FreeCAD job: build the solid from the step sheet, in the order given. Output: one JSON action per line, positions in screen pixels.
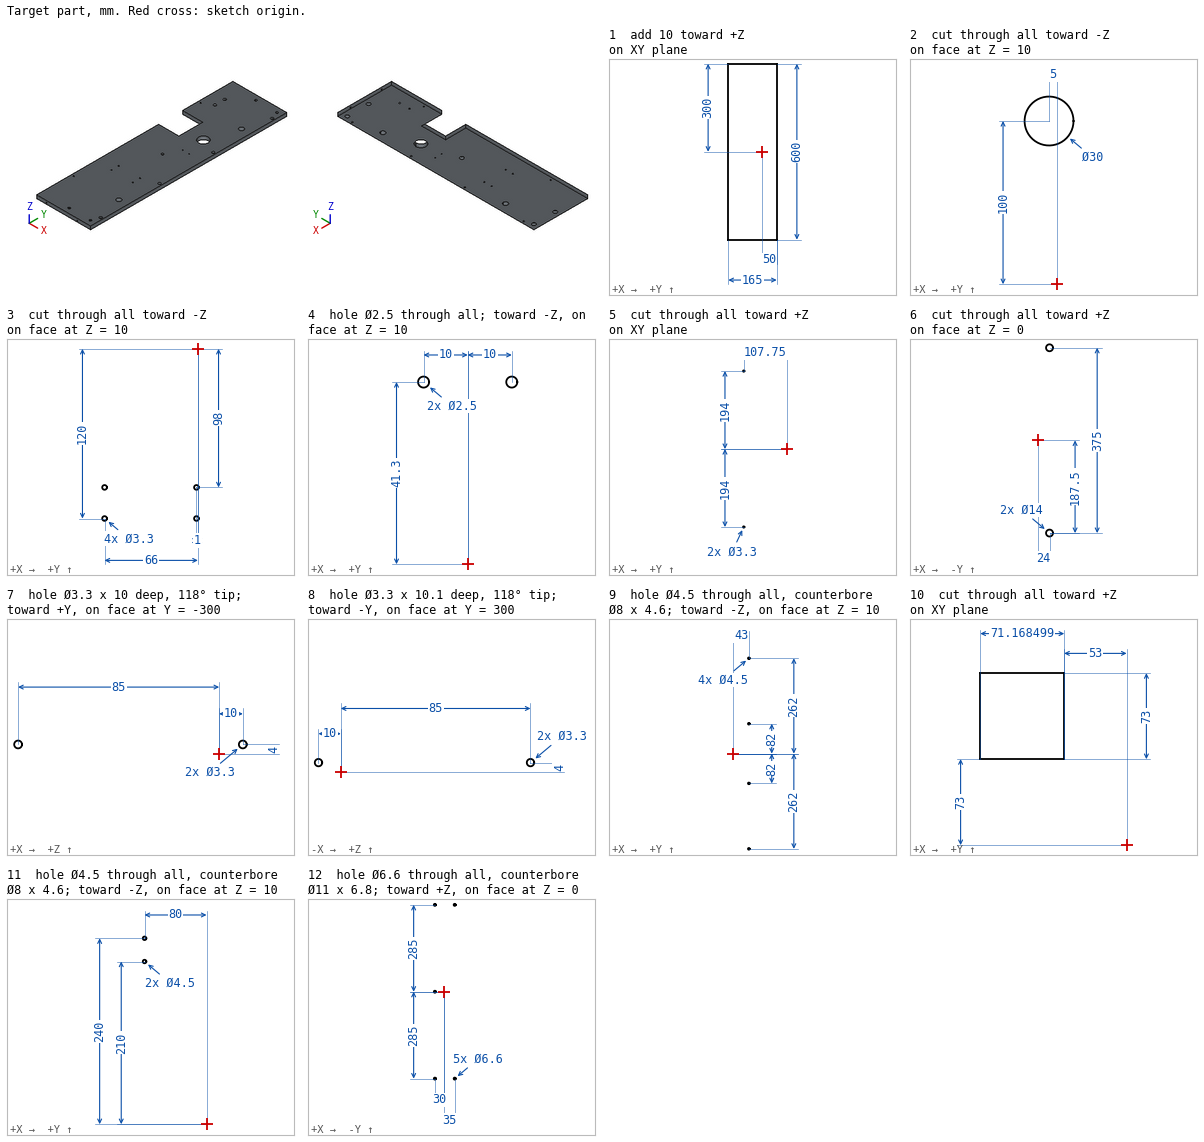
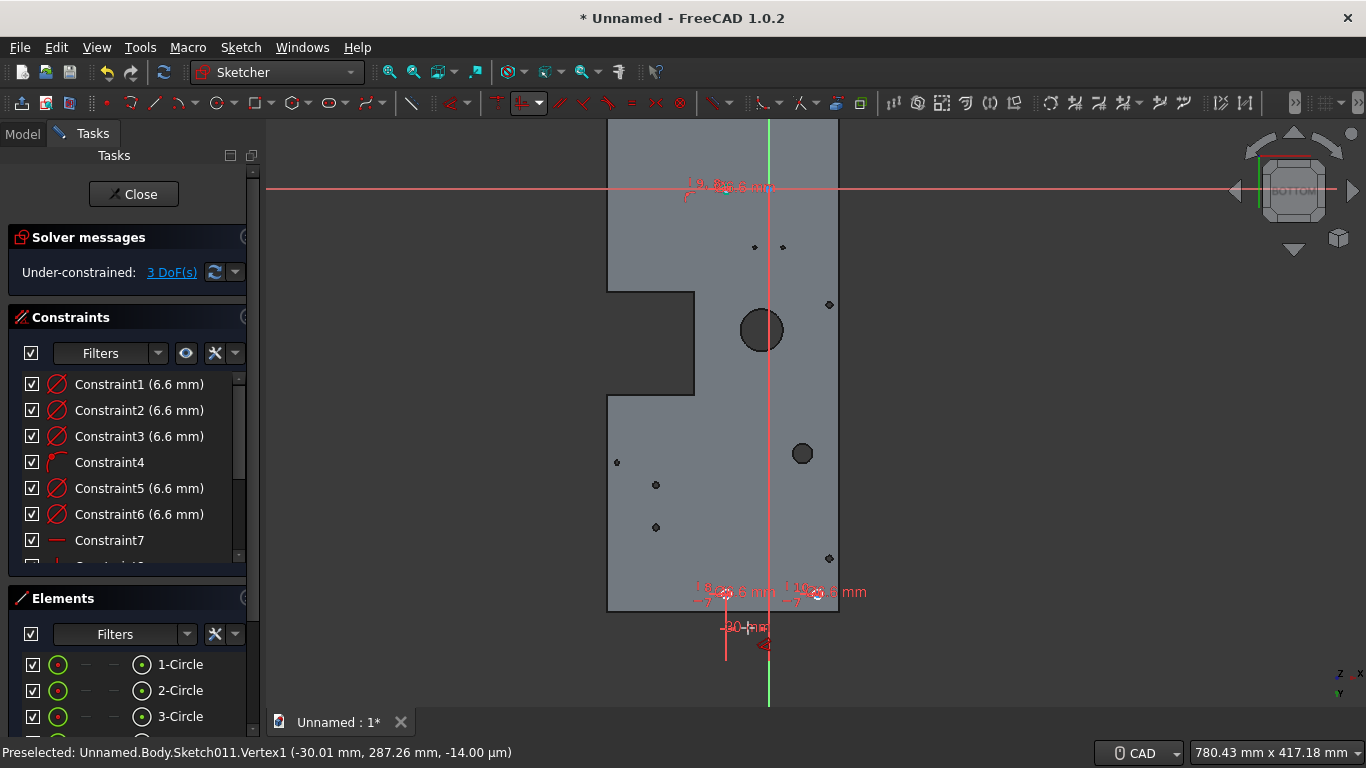
{"action": "left_click", "coordinate": [818, 594]}
{"action": "left_click", "coordinate": [793, 155]}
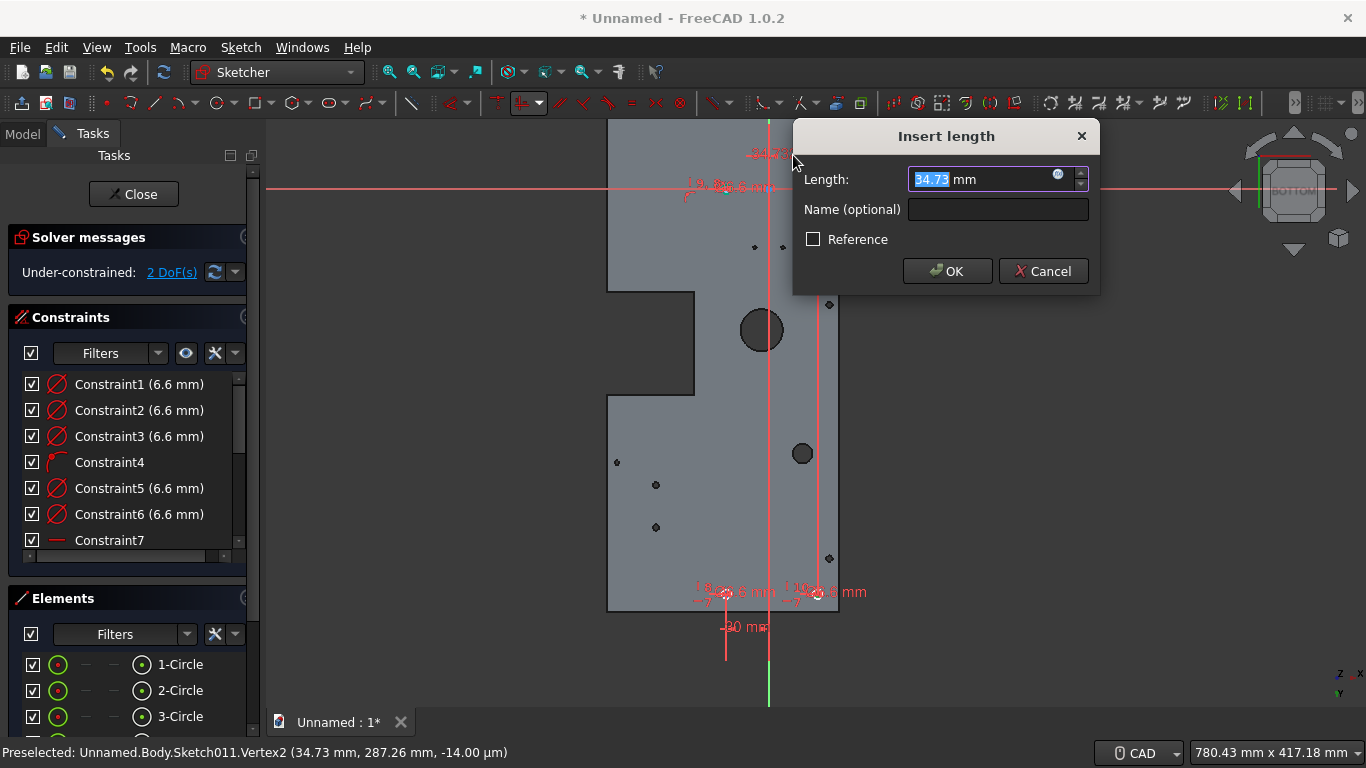
{"action": "type", "text": "35"}
{"action": "key", "text": "Return"}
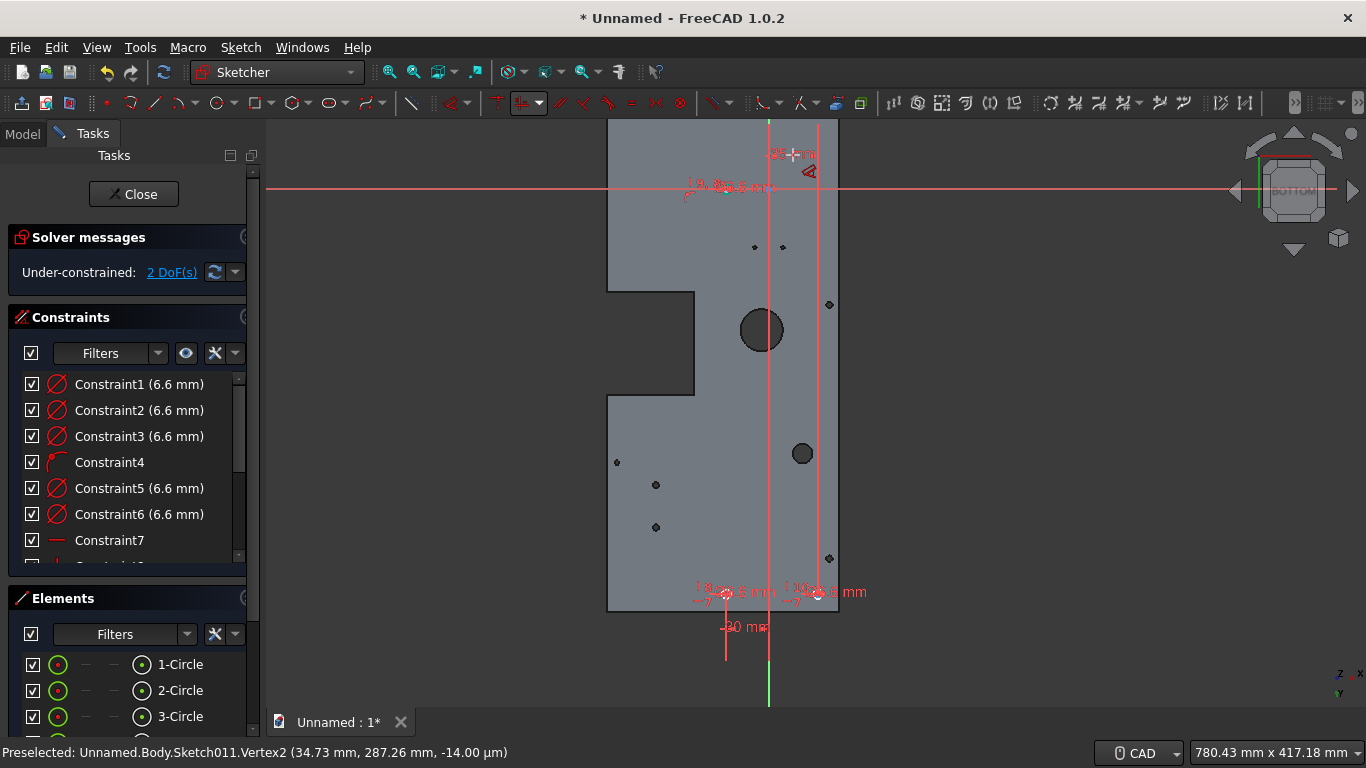
{"action": "left_click", "coordinate": [726, 594]}
{"action": "left_click", "coordinate": [692, 392]}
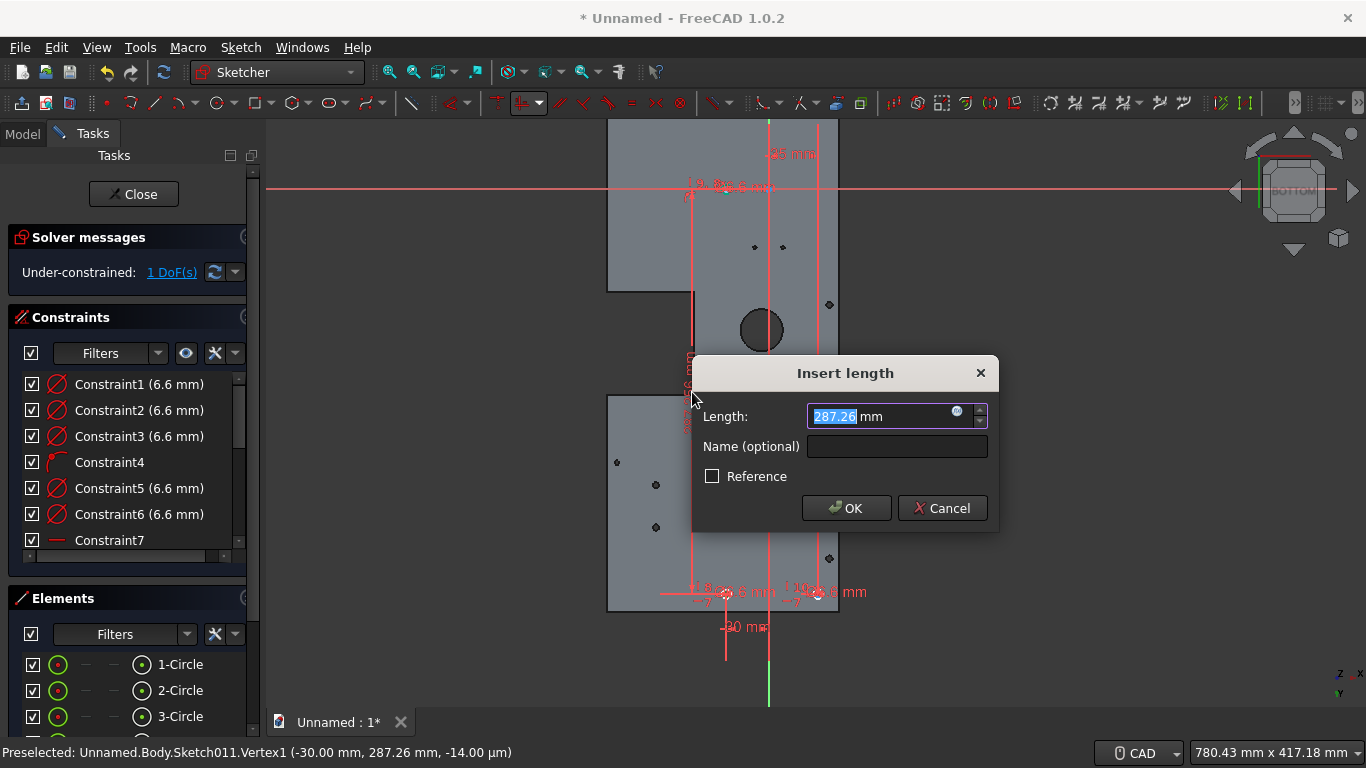
{"action": "type", "text": "285"}
{"action": "key", "text": "Return"}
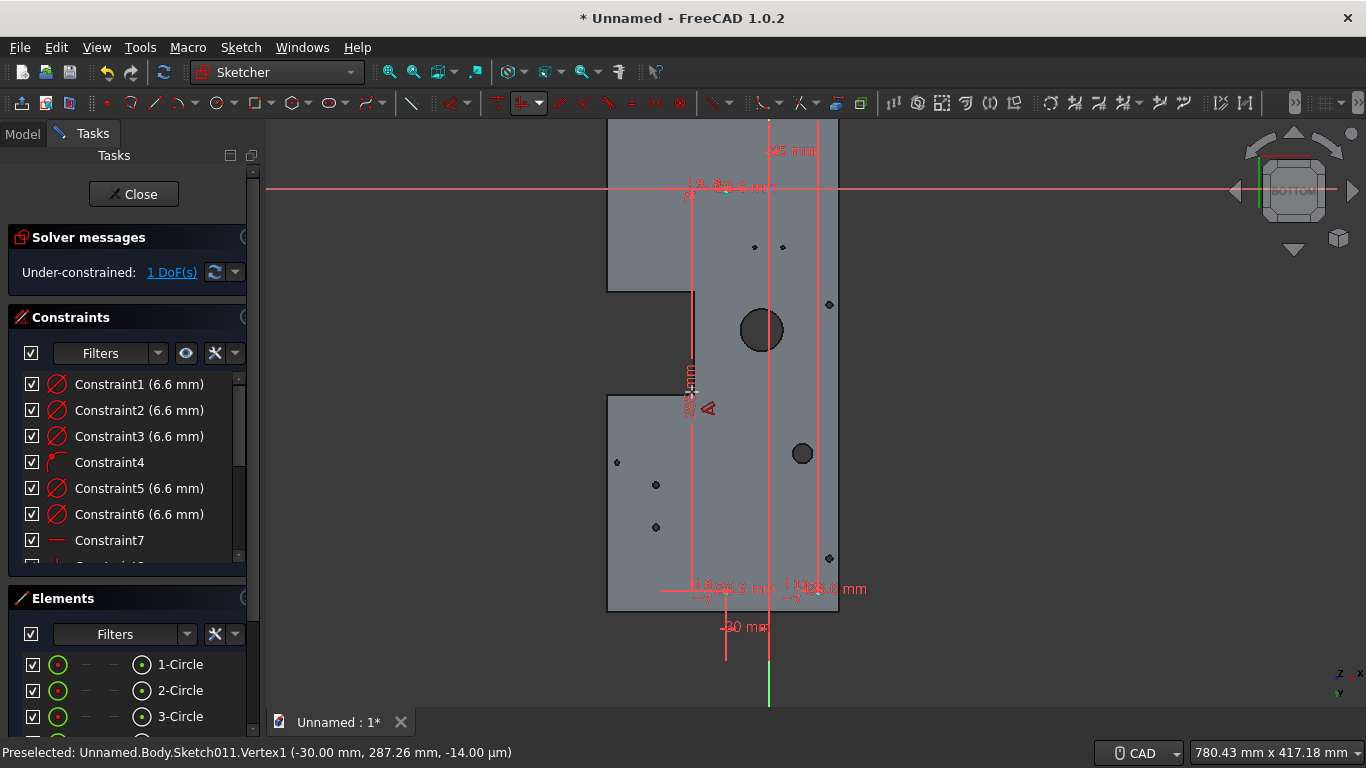
{"action": "scroll", "coordinate": [727, 596], "scroll_direction": "down", "scroll_amount": 4}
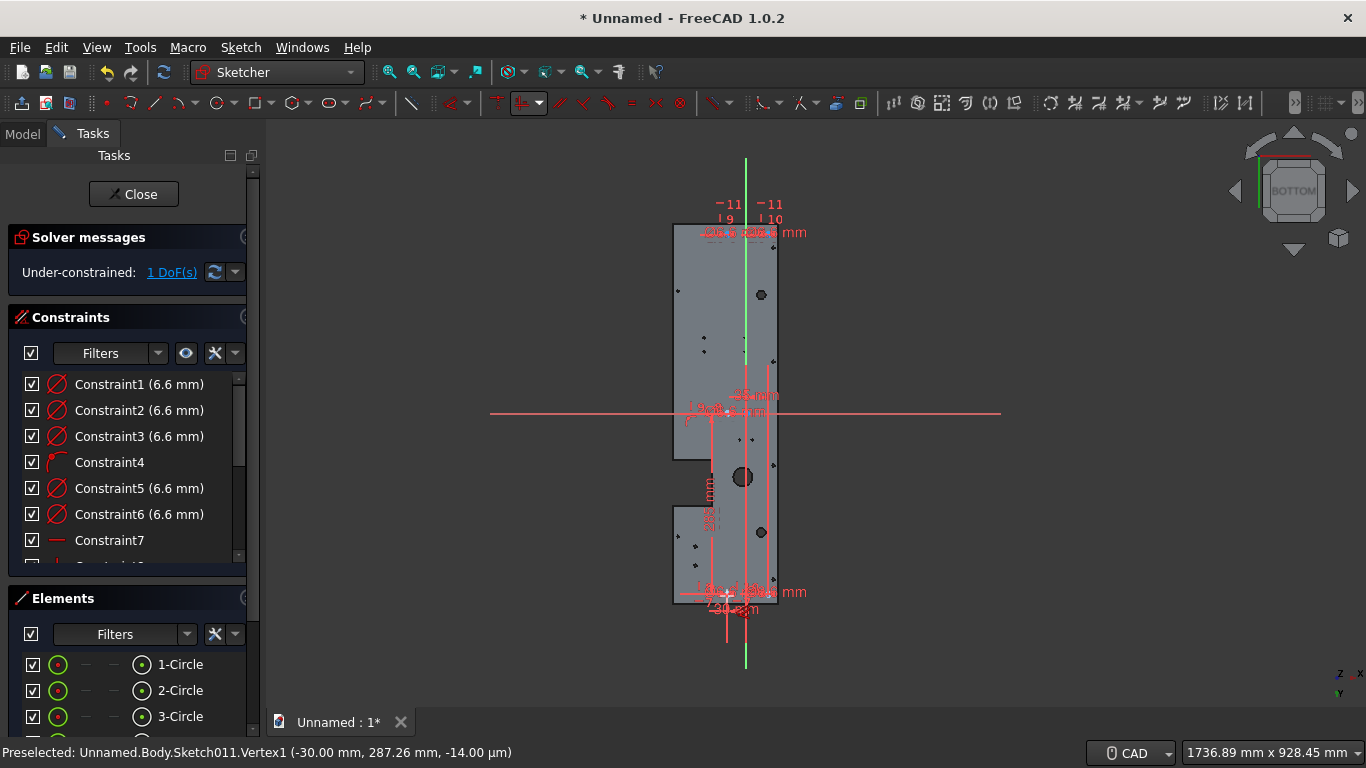
{"action": "left_click", "coordinate": [727, 235]}
{"action": "left_click", "coordinate": [693, 324]}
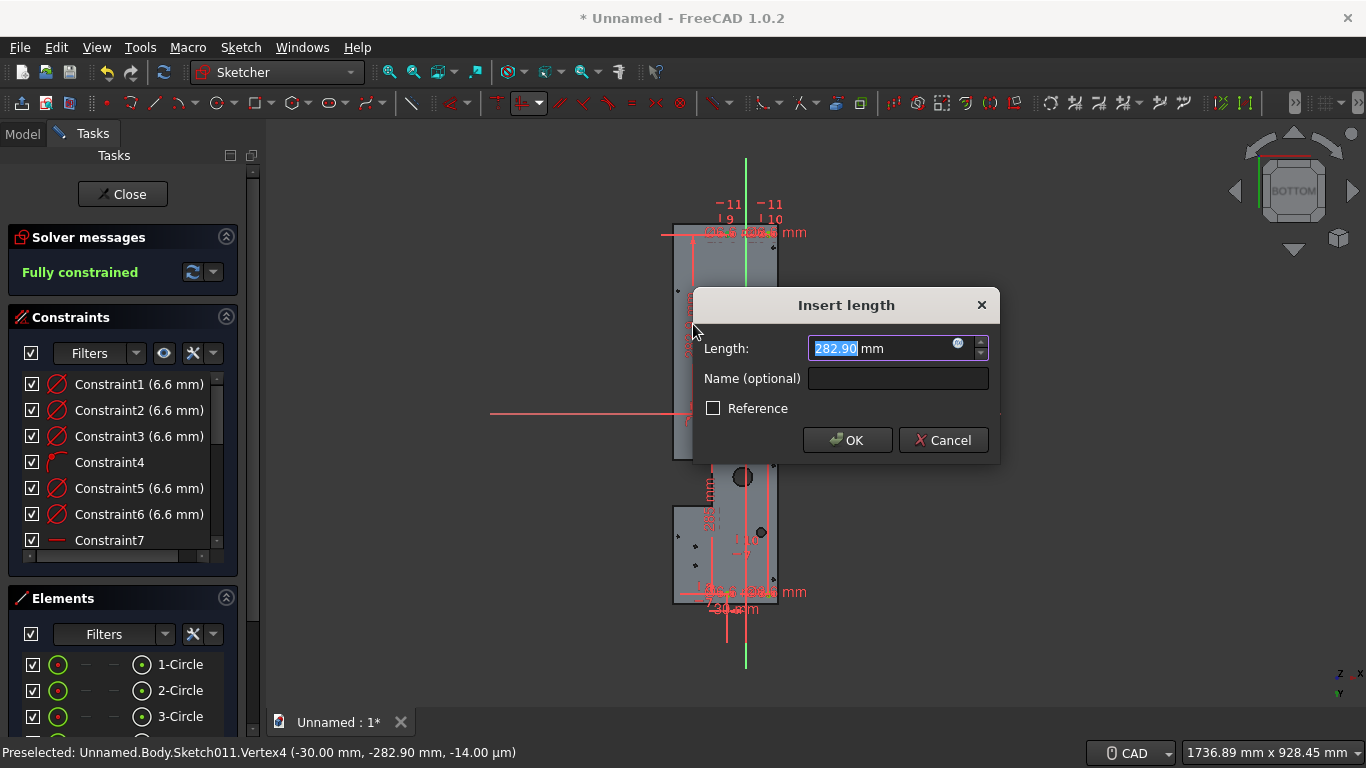
{"action": "type", "text": "285"}
{"action": "key", "text": "Return"}
{"action": "key", "text": "Escape"}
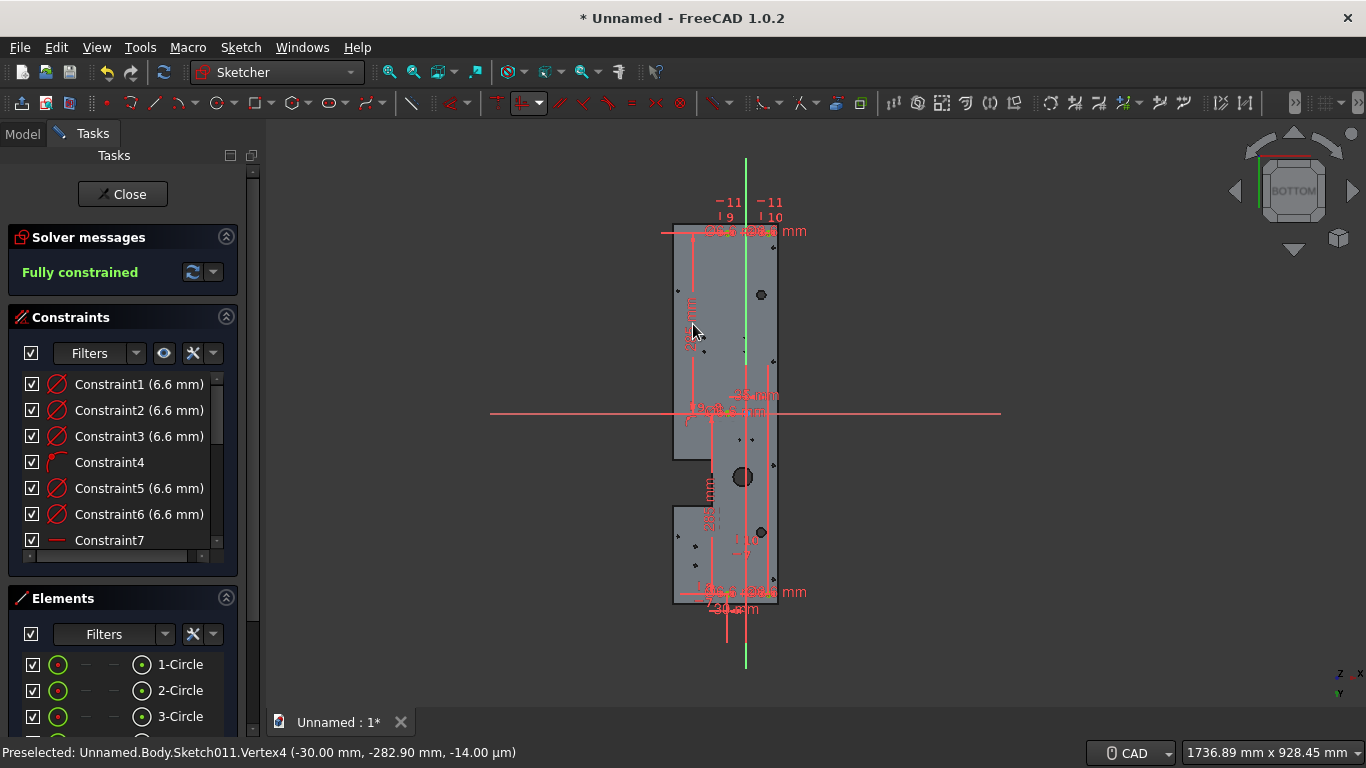
{"action": "left_click", "coordinate": [123, 194]}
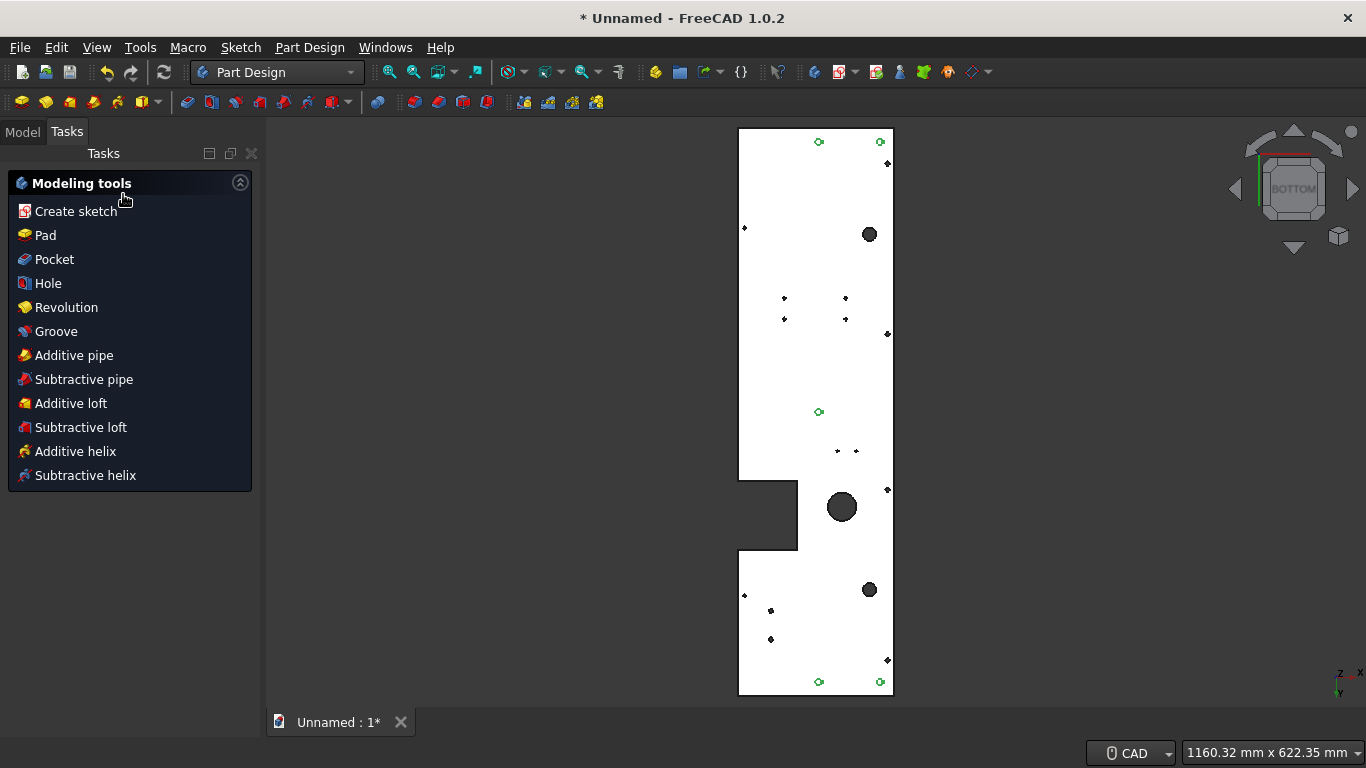
{"action": "left_click", "coordinate": [212, 102]}